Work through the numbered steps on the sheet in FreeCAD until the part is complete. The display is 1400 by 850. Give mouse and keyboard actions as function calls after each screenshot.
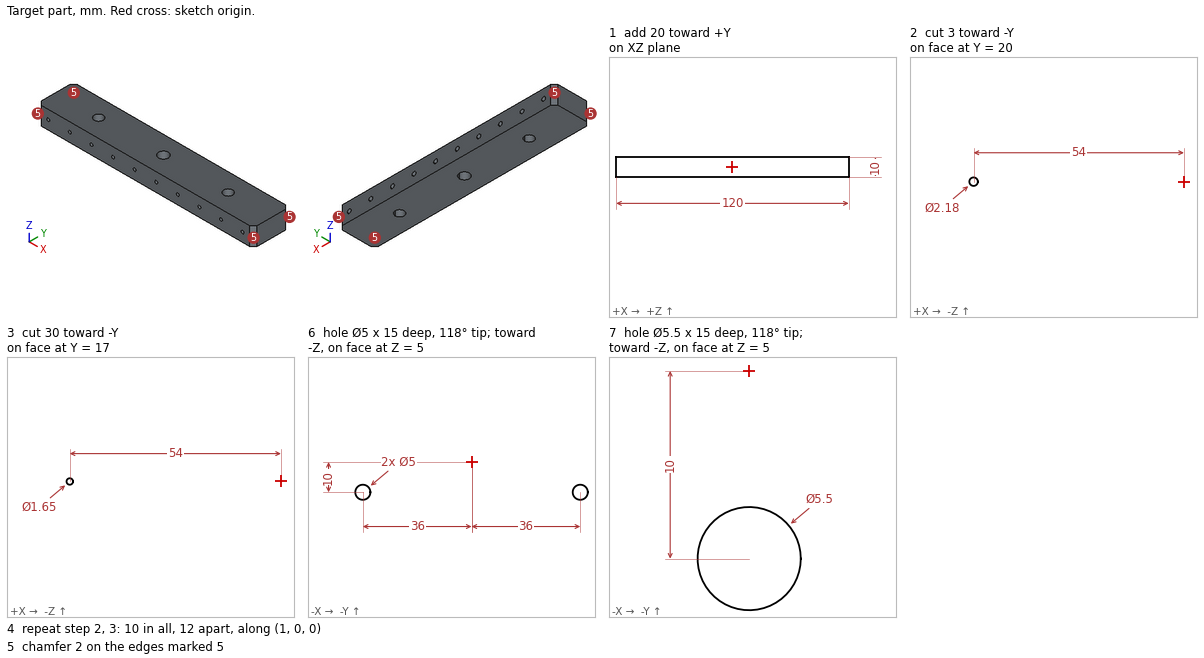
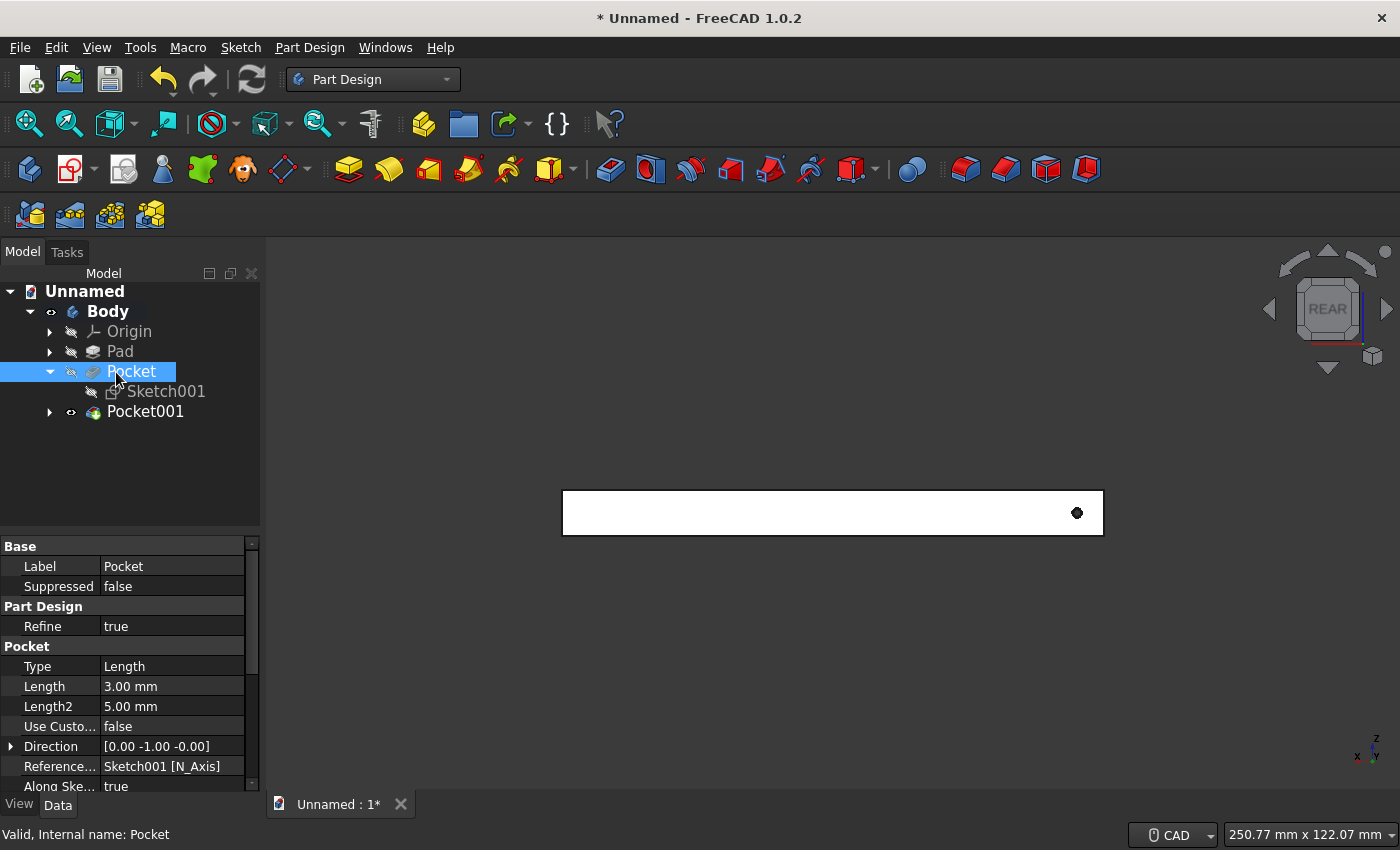
click(116, 412, ctrl)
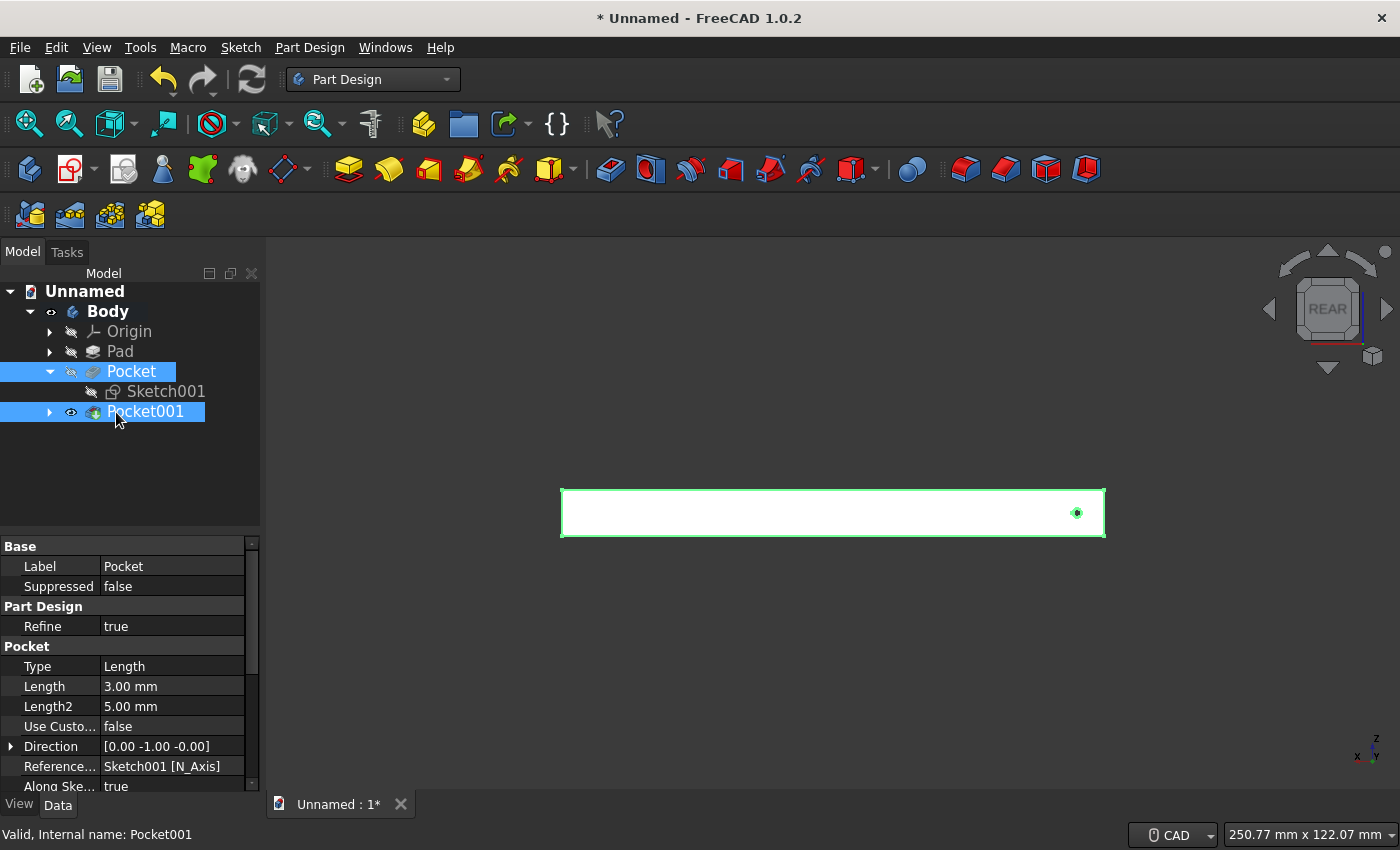
click(70, 214)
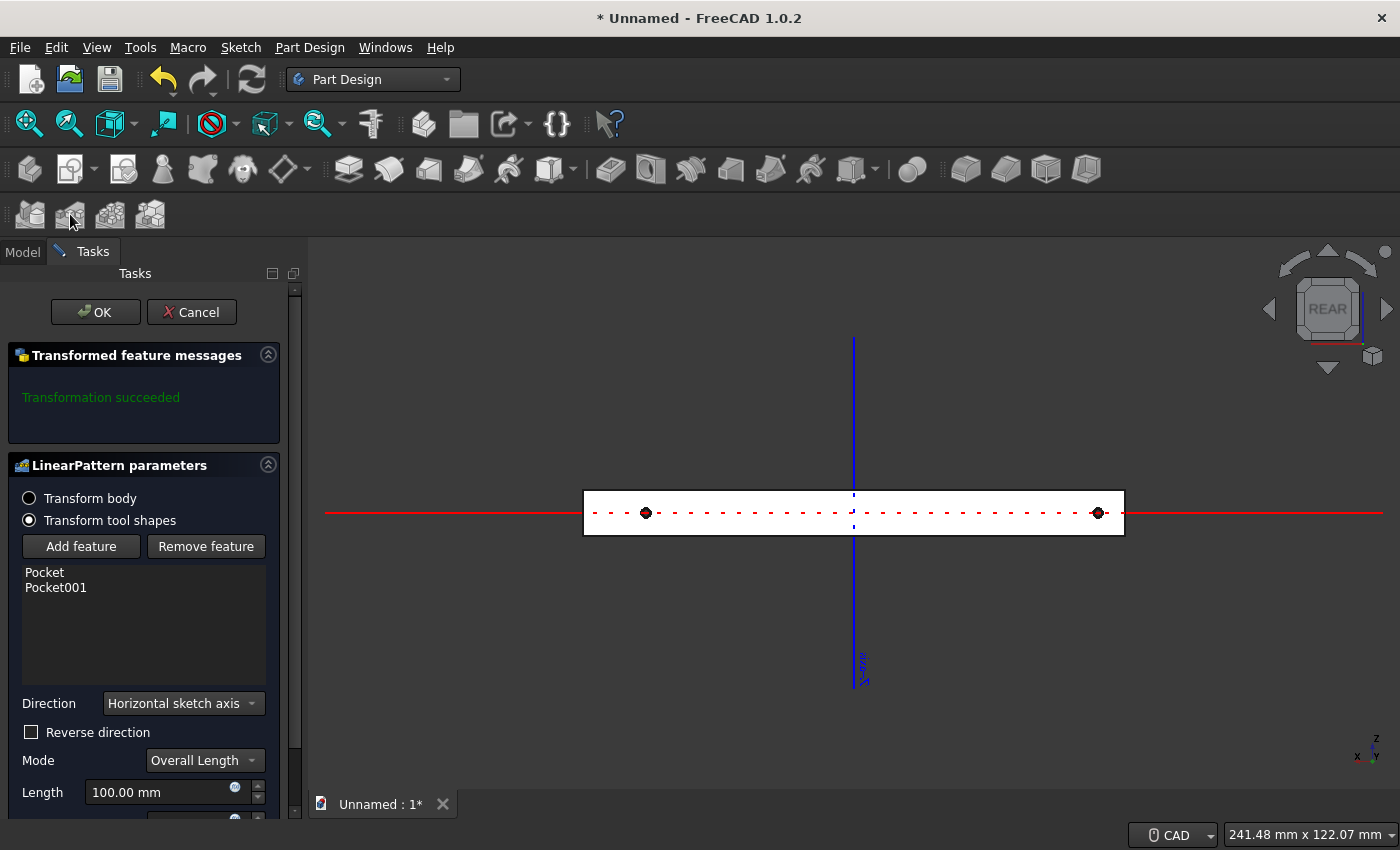
click(184, 704)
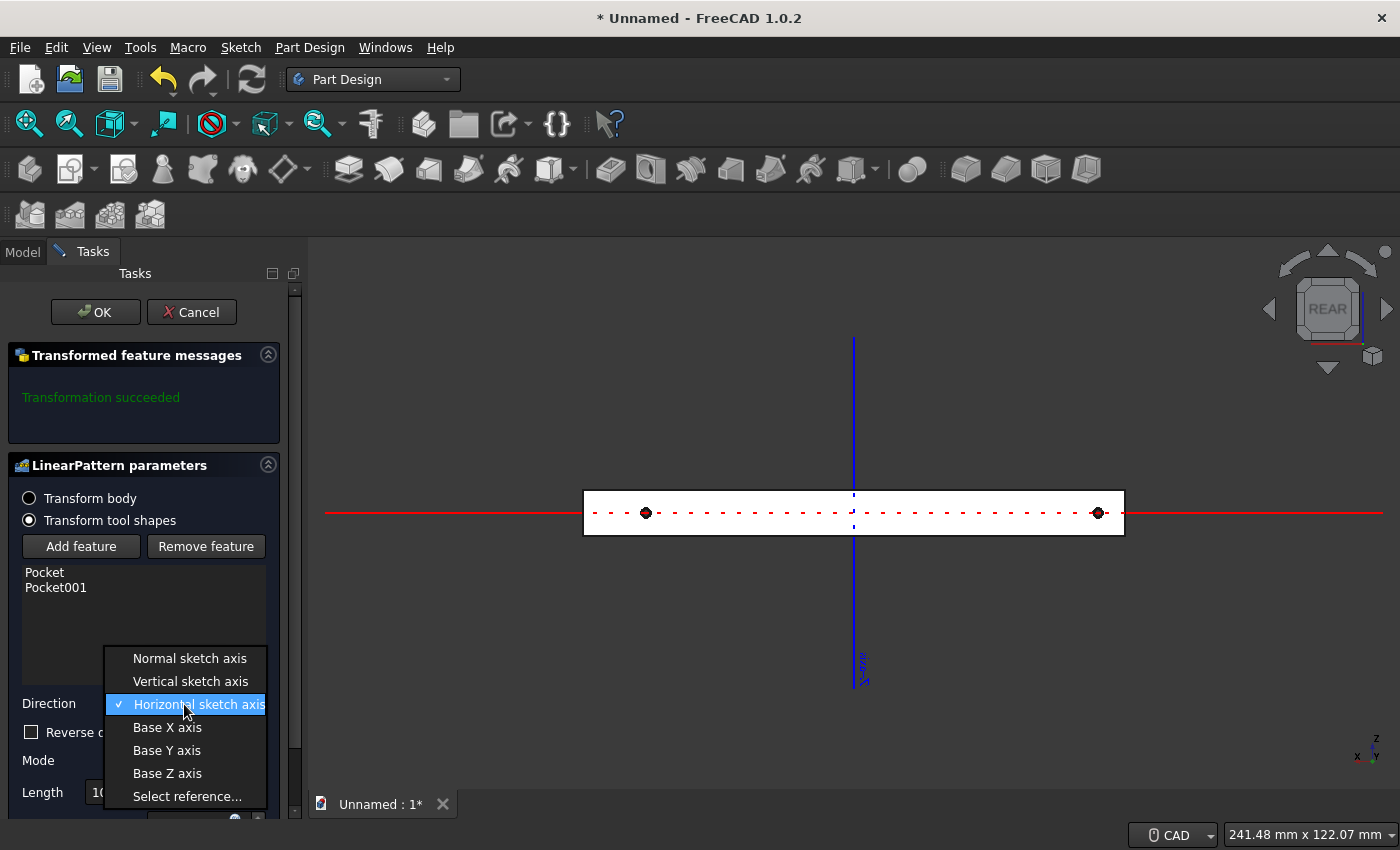
click(184, 728)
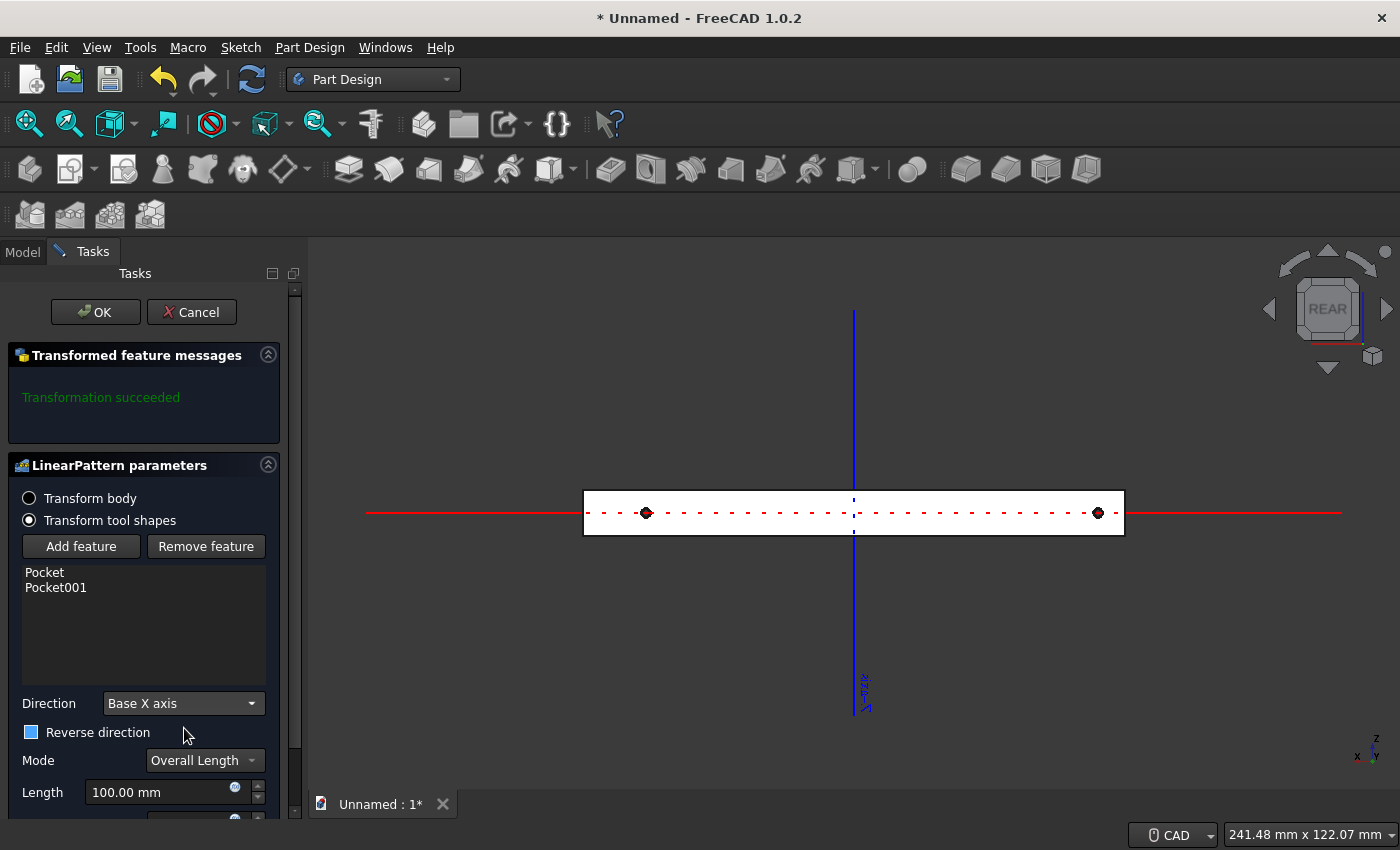
click(206, 760)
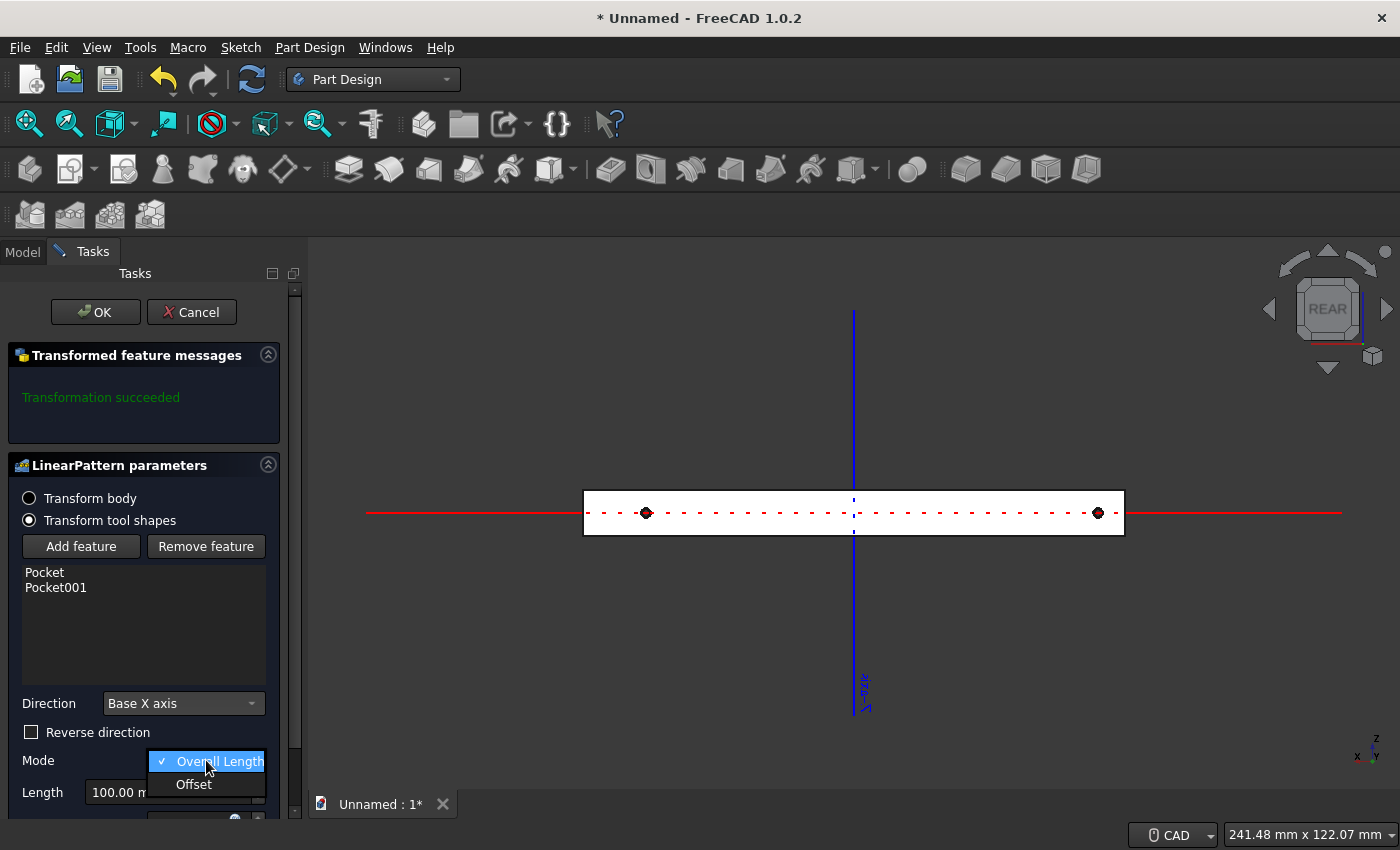
click(206, 784)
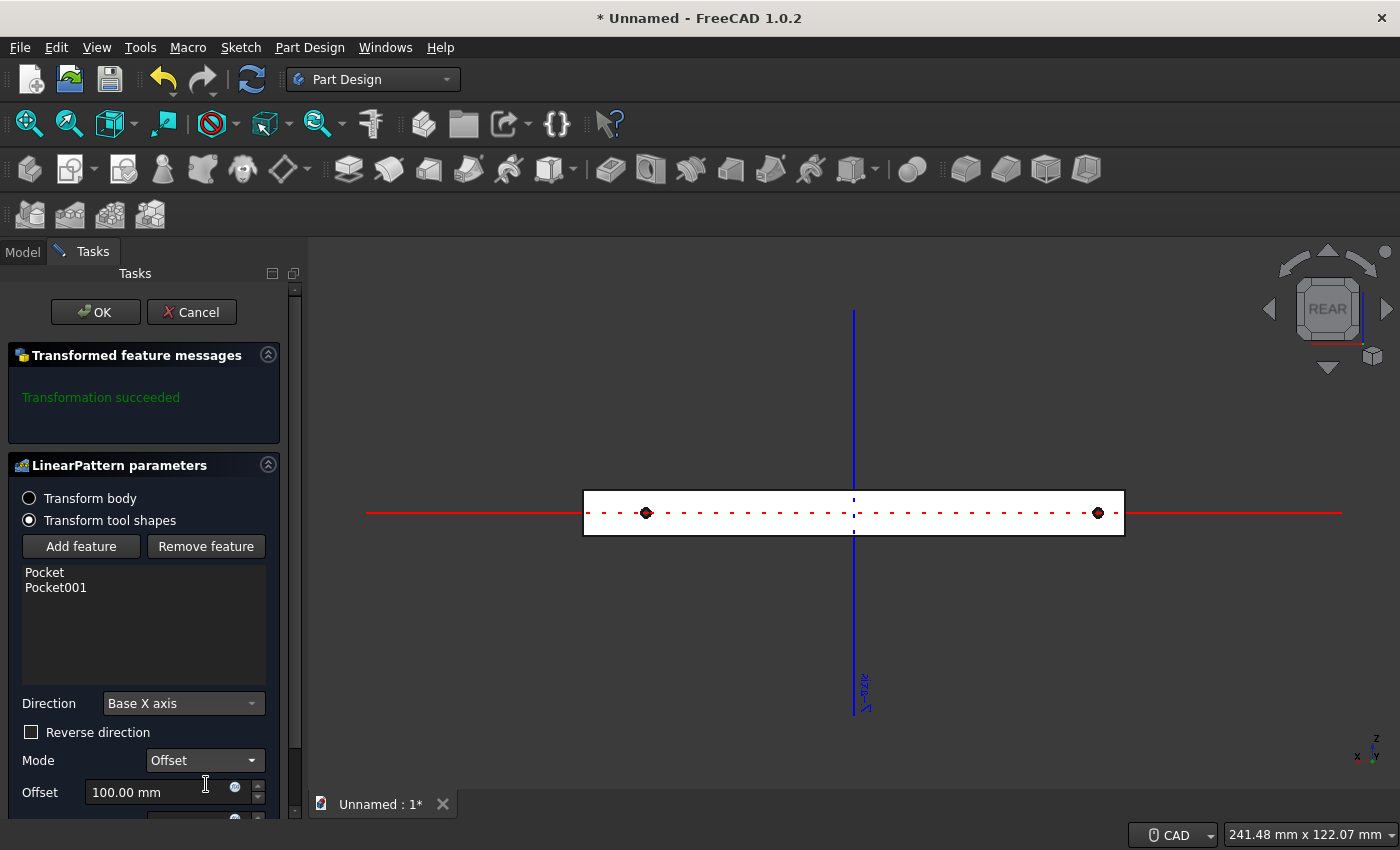
triple_click(168, 792)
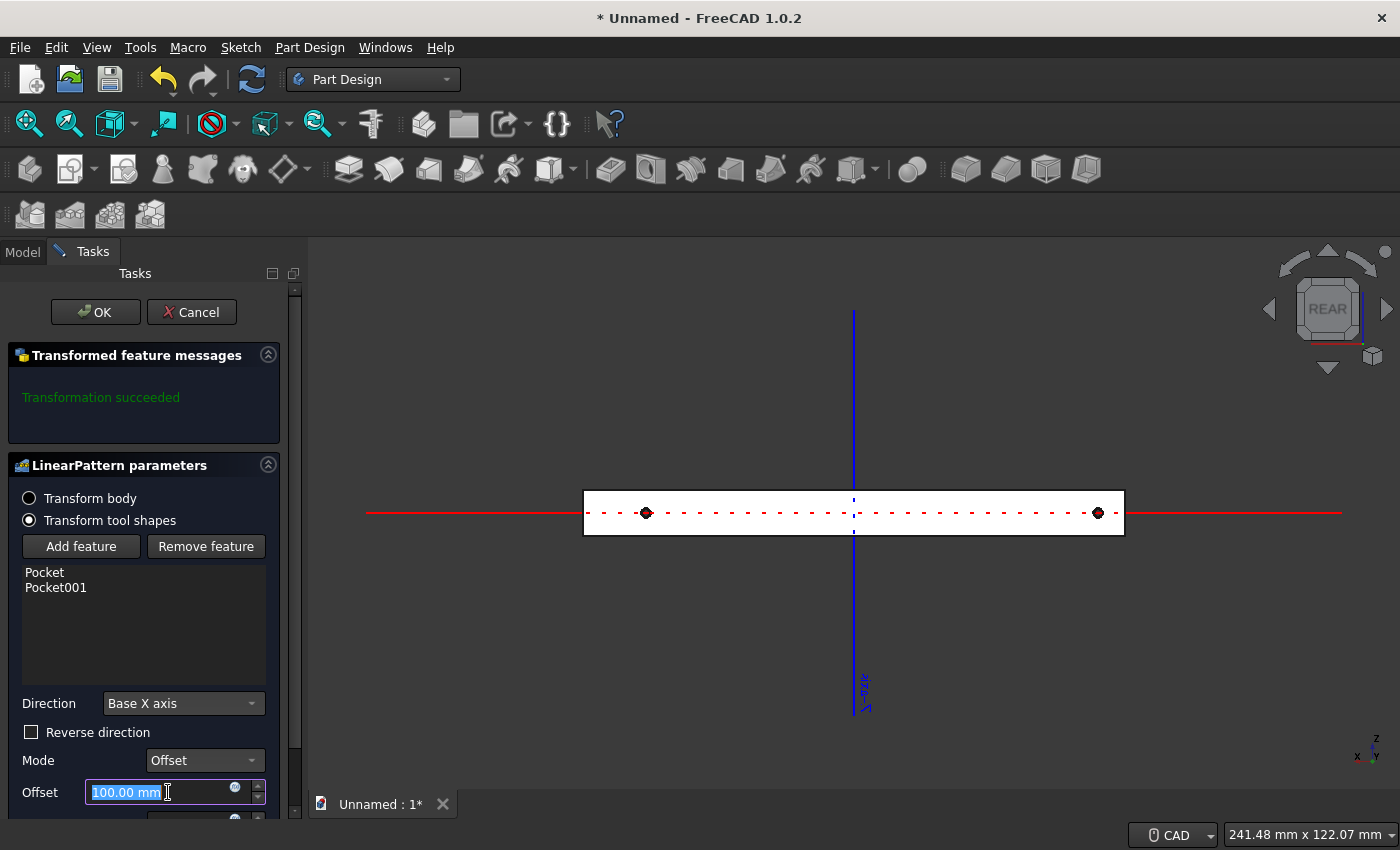
text(12)
key(Tab)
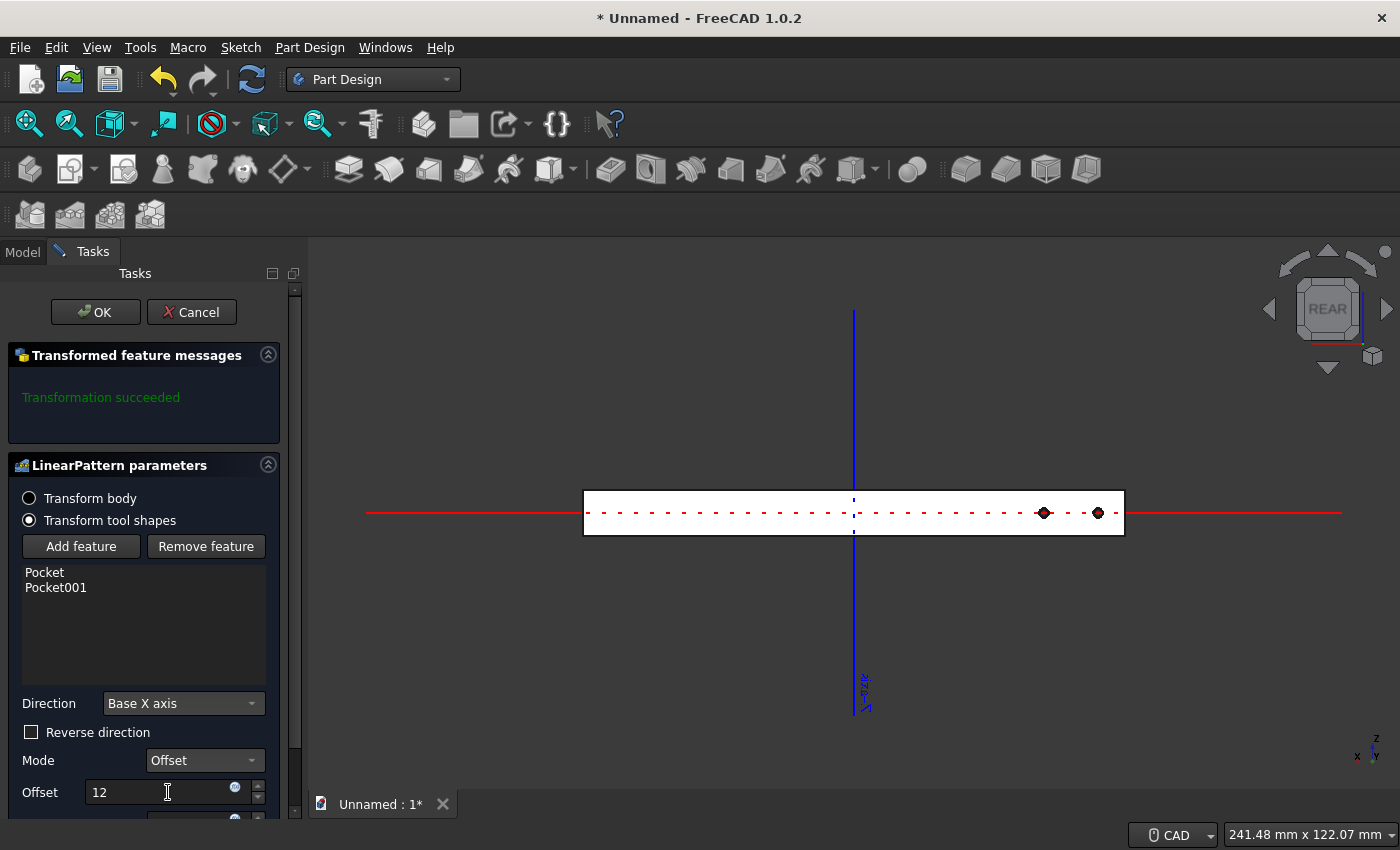
scroll(295, 550, down, 2)